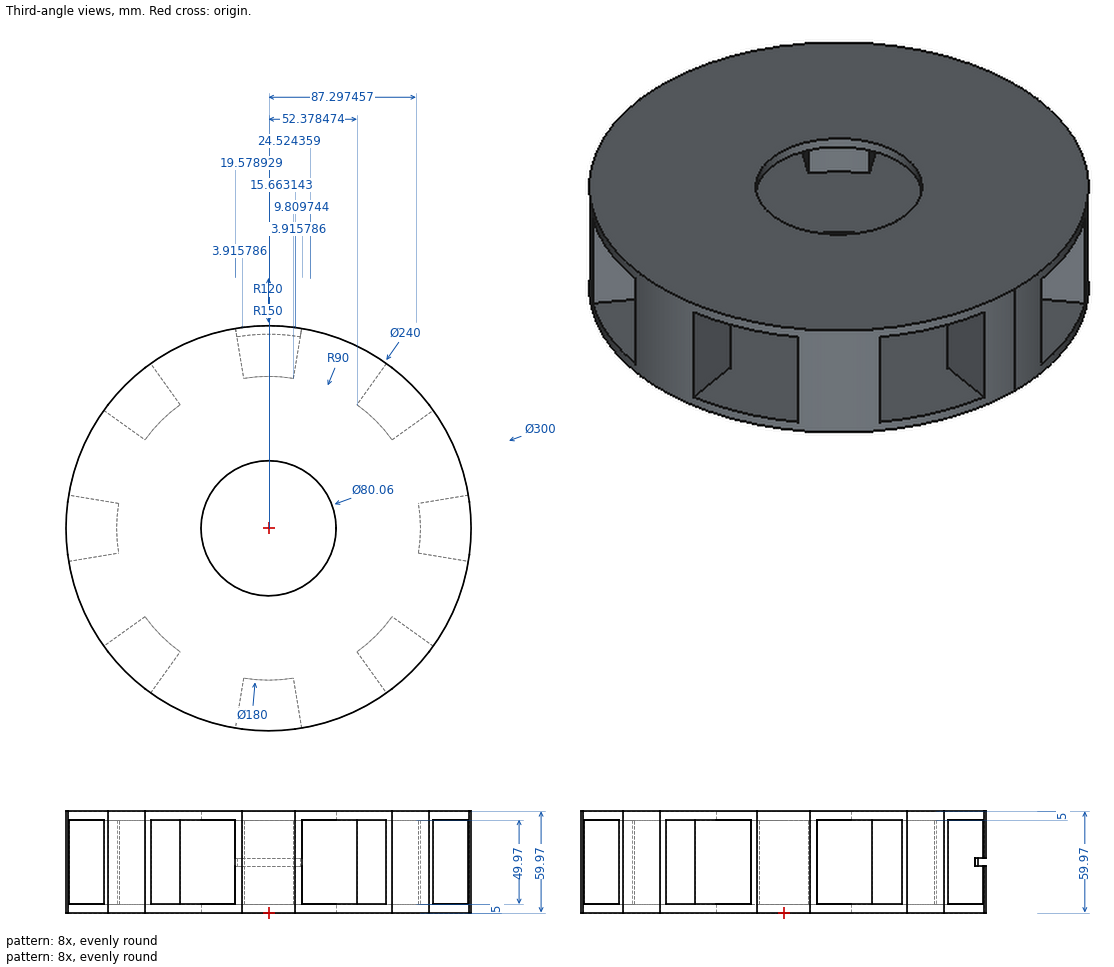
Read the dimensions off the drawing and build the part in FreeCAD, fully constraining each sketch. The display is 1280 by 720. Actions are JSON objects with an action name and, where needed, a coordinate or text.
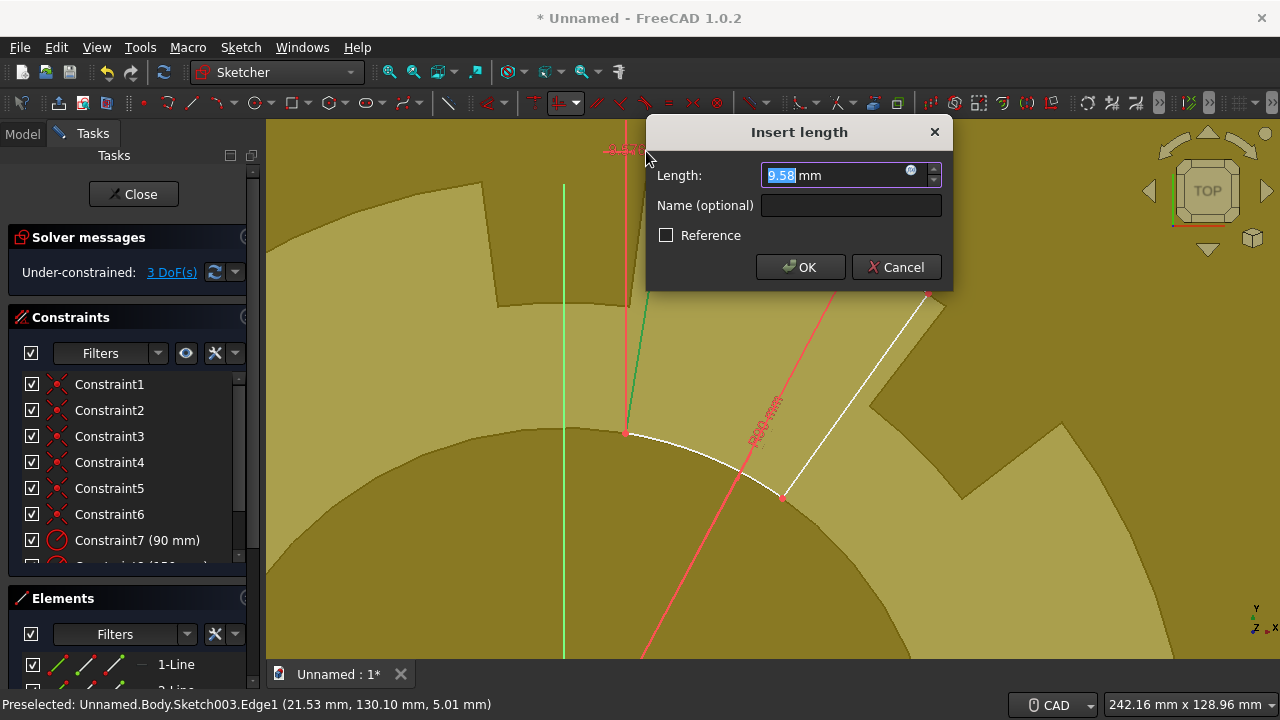
{"action": "type", "text": "9.809744"}
{"action": "key", "text": "Return"}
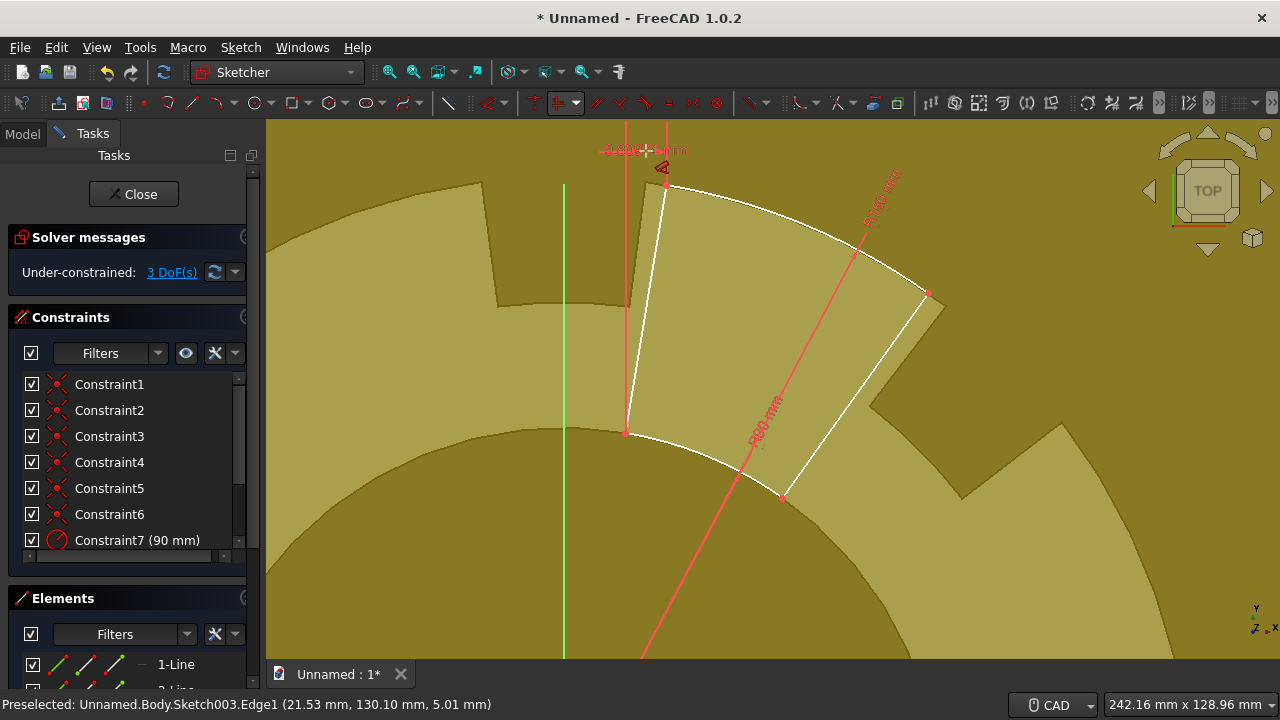
{"action": "left_click", "coordinate": [667, 185]}
{"action": "left_click", "coordinate": [591, 151]}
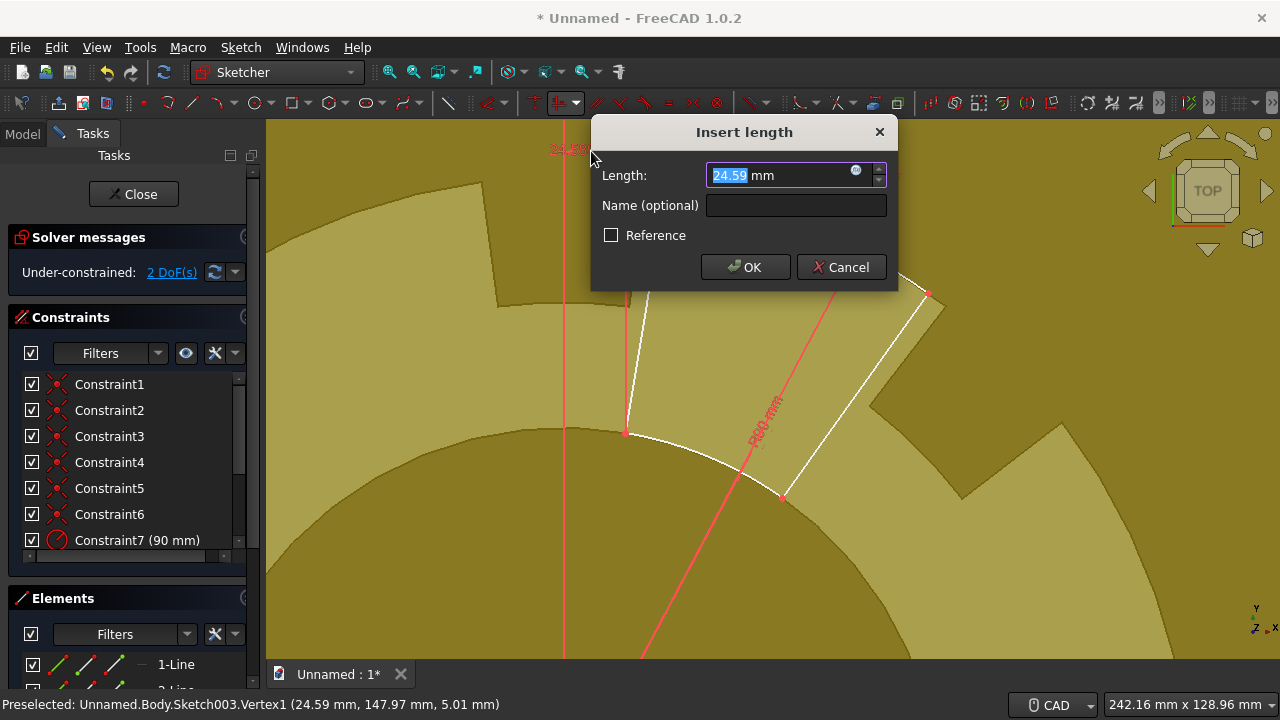
{"action": "type", "text": "24.524359"}
{"action": "key", "text": "Return"}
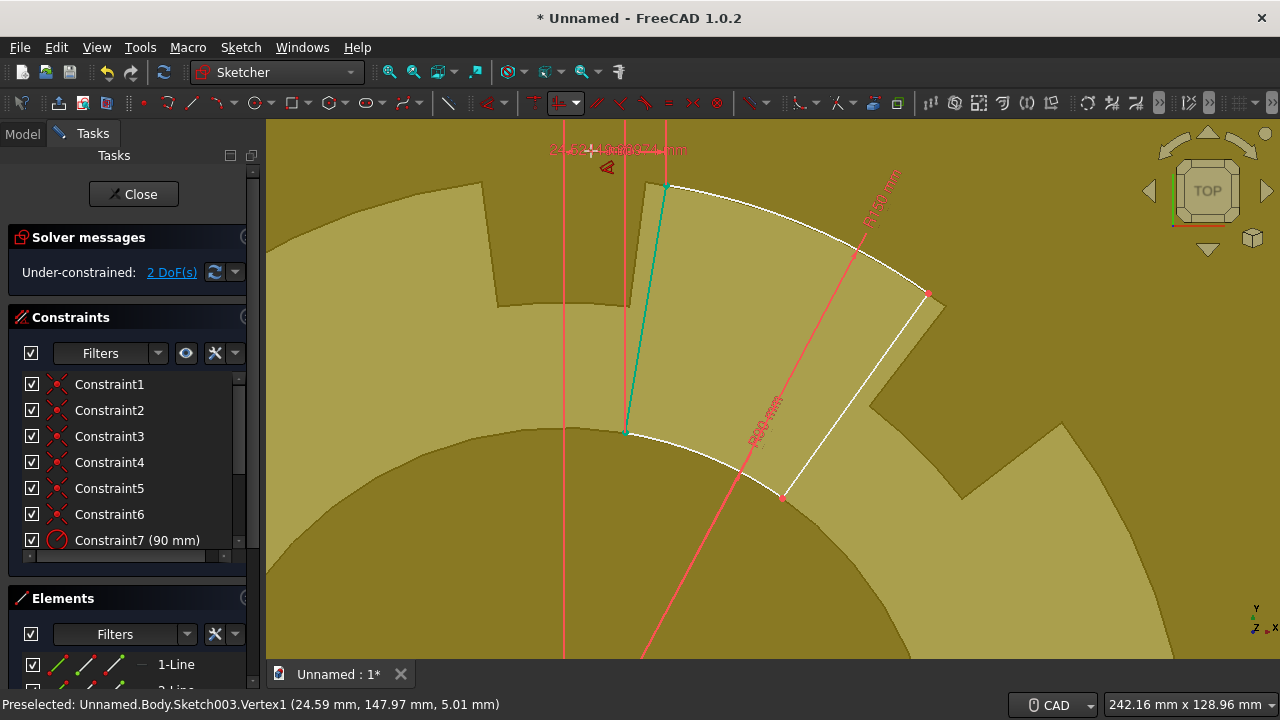
{"action": "left_click", "coordinate": [783, 498]}
{"action": "left_click", "coordinate": [673, 464]}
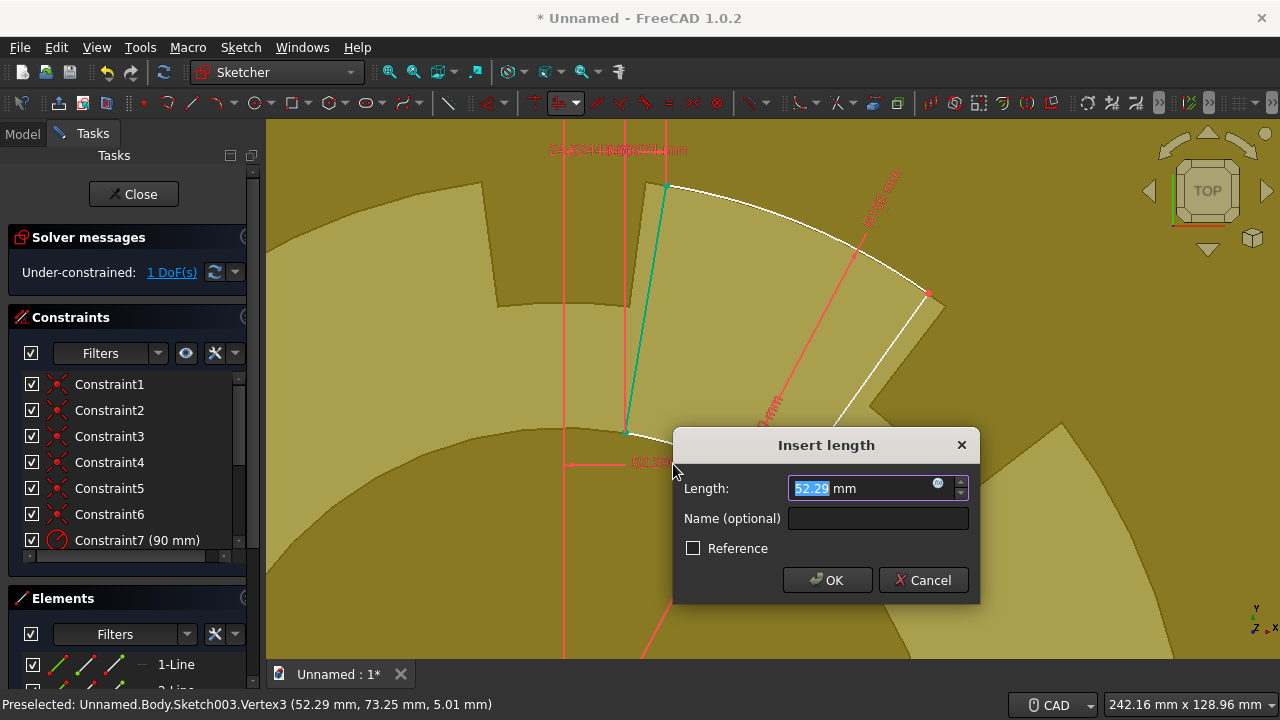
{"action": "type", "text": "52.378474"}
{"action": "key", "text": "Return"}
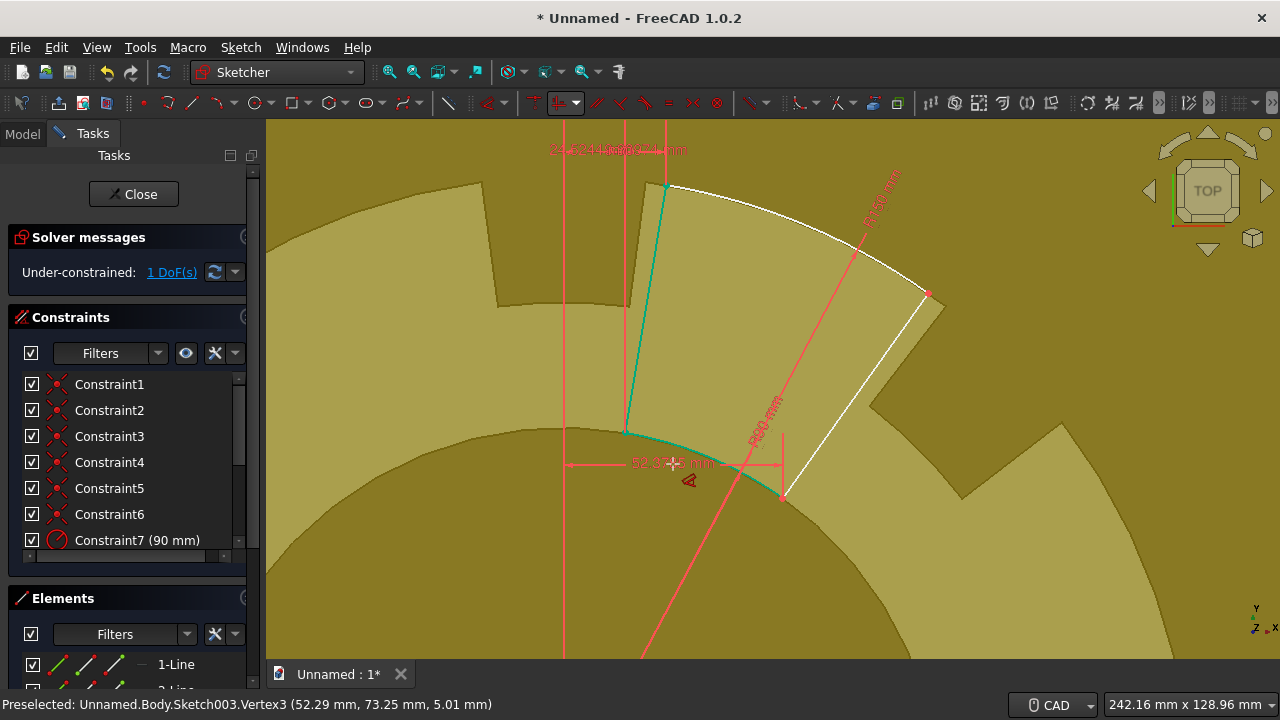
{"action": "left_click", "coordinate": [928, 293]}
{"action": "left_click", "coordinate": [746, 259]}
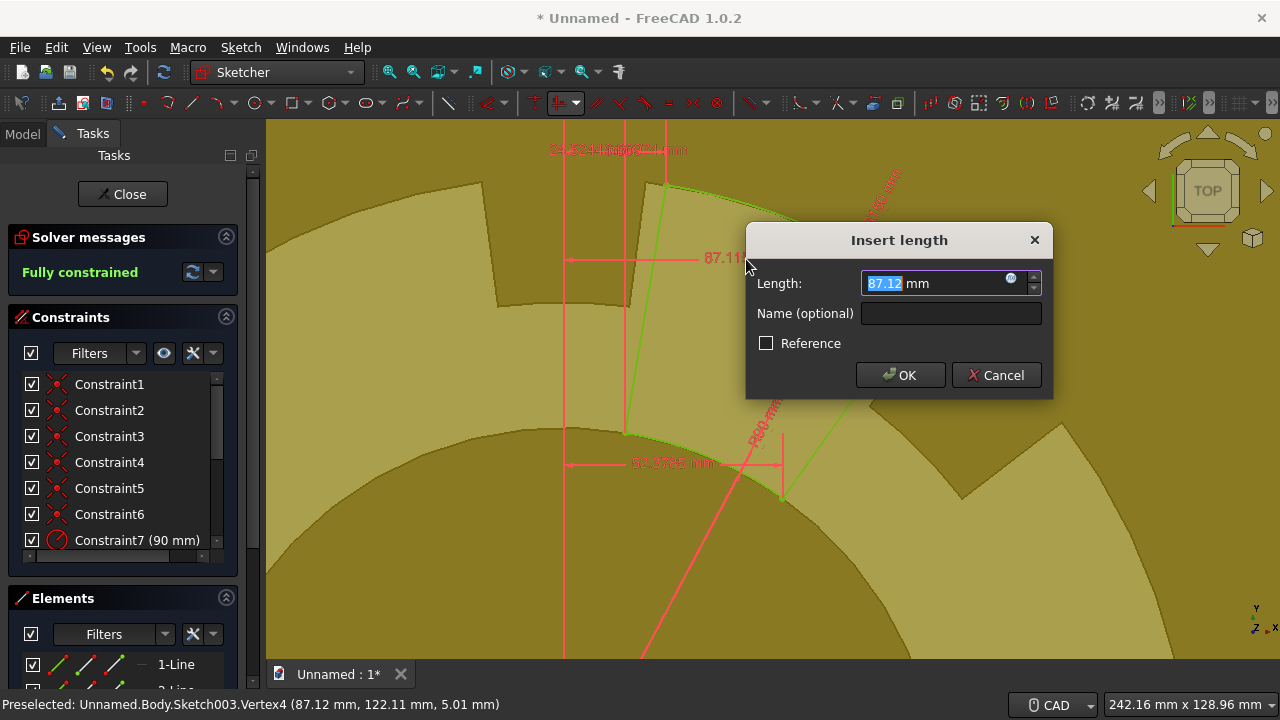
{"action": "type", "text": "87.297457"}
{"action": "key", "text": "Return"}
{"action": "key", "text": "Escape"}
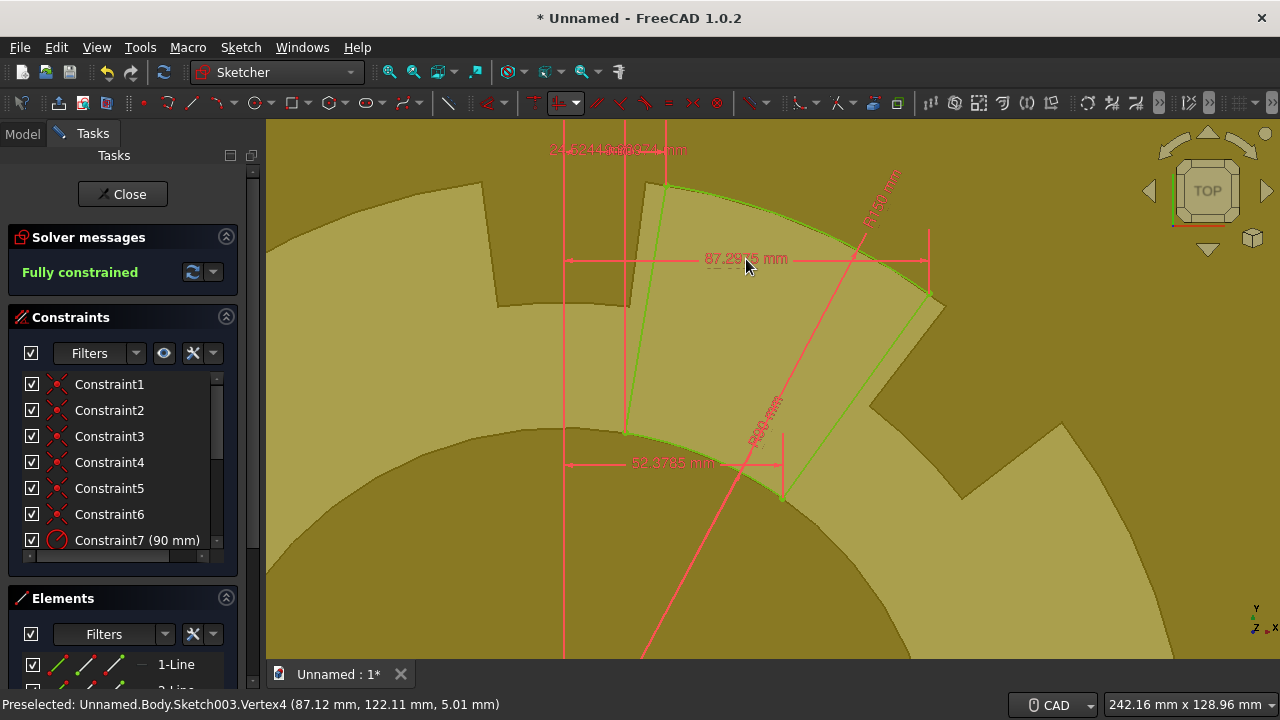
{"action": "left_click", "coordinate": [123, 194]}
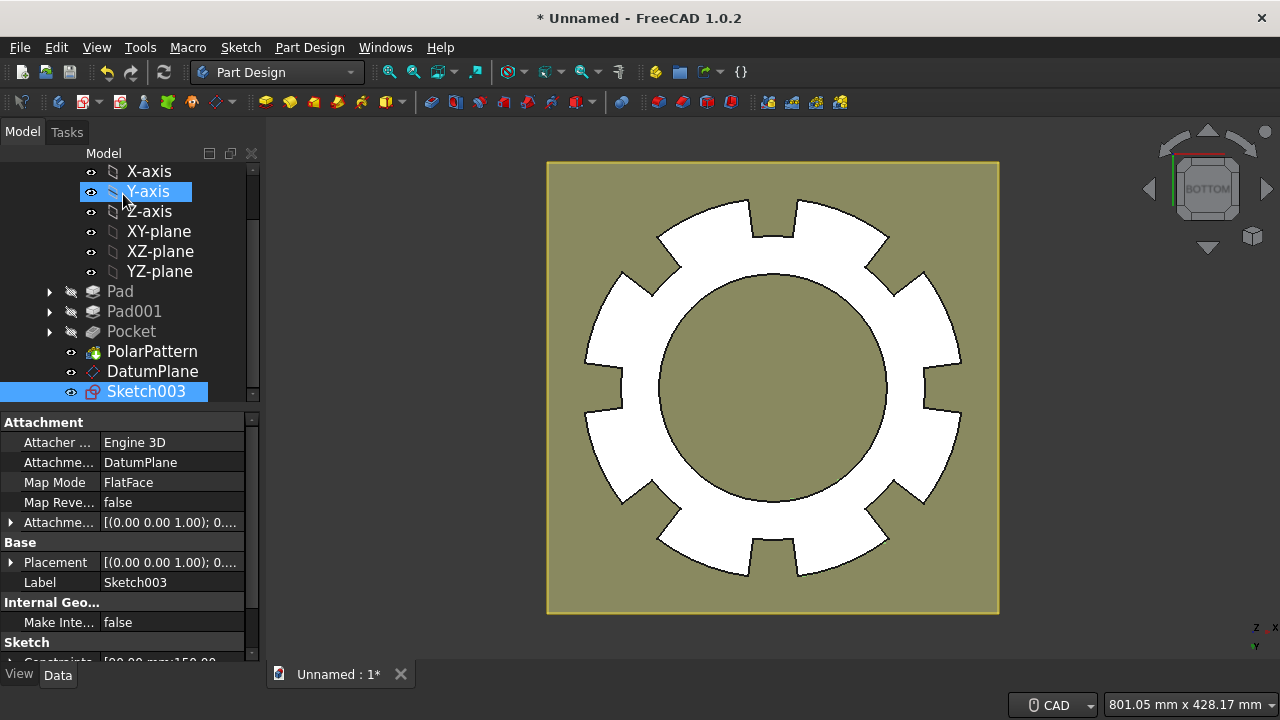
{"action": "left_click", "coordinate": [432, 102]}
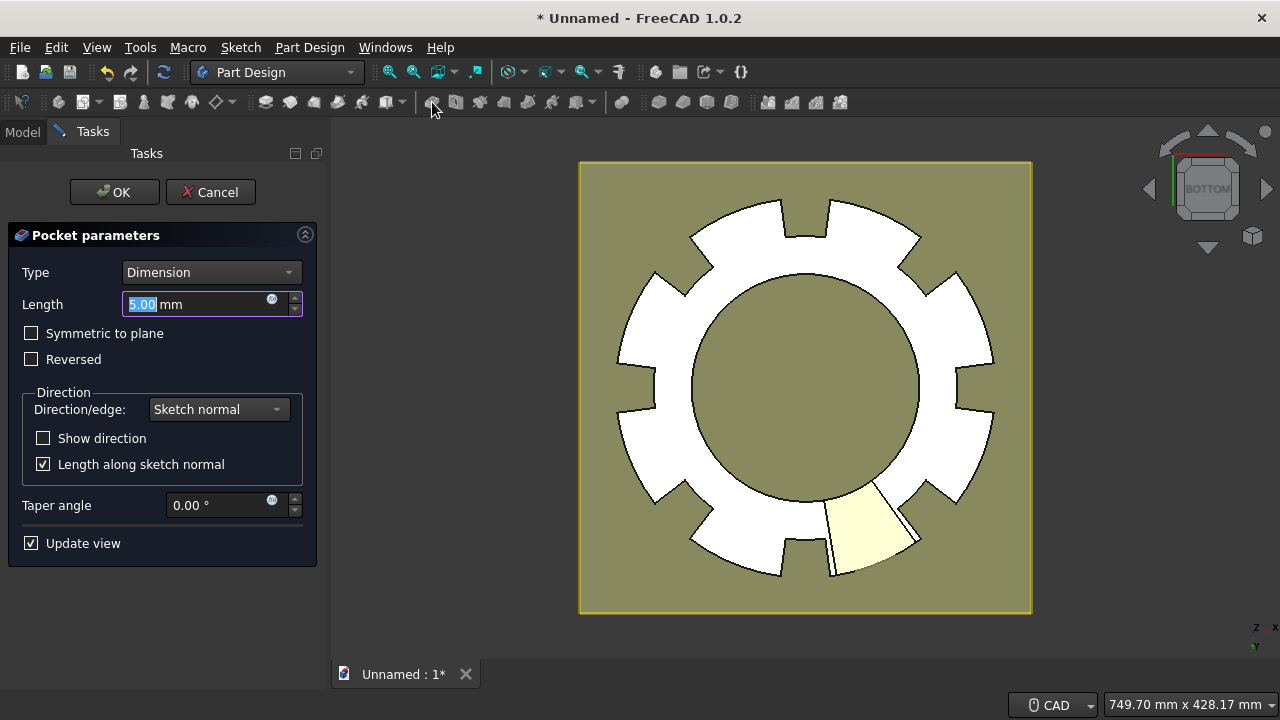
{"action": "type", "text": "49.97"}
{"action": "key", "text": "Tab"}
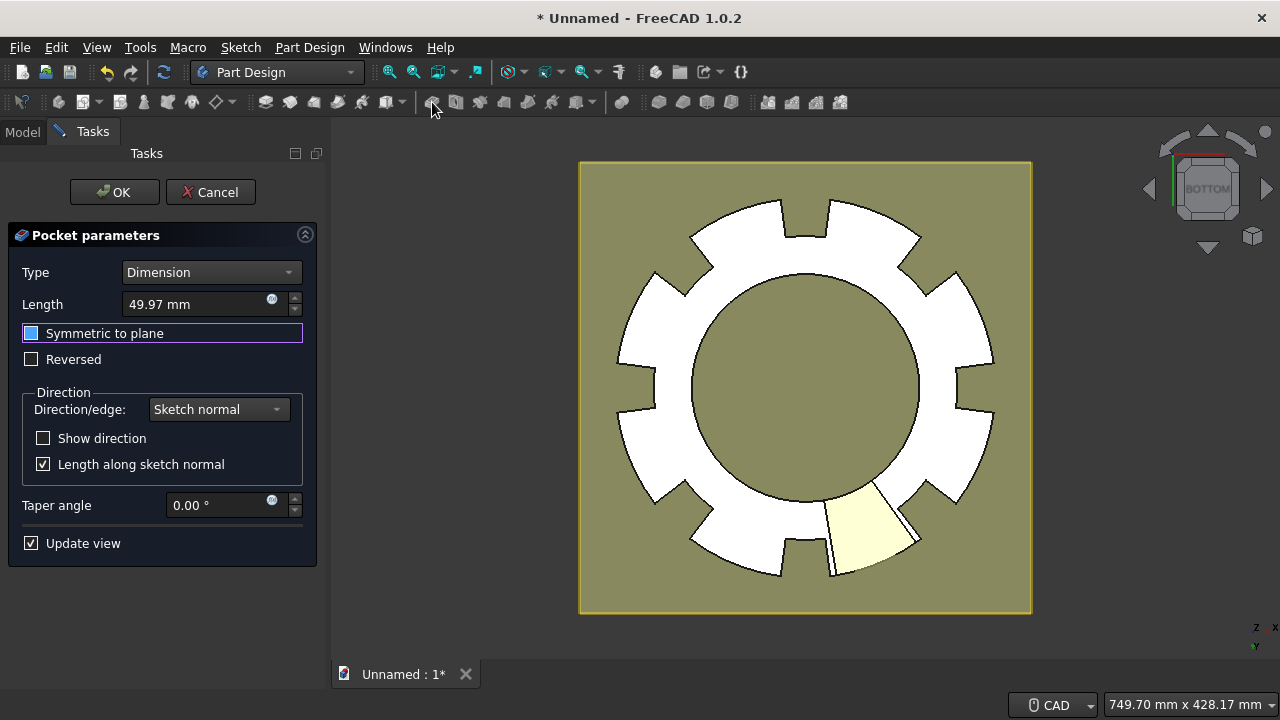
{"action": "left_click", "coordinate": [30, 359]}